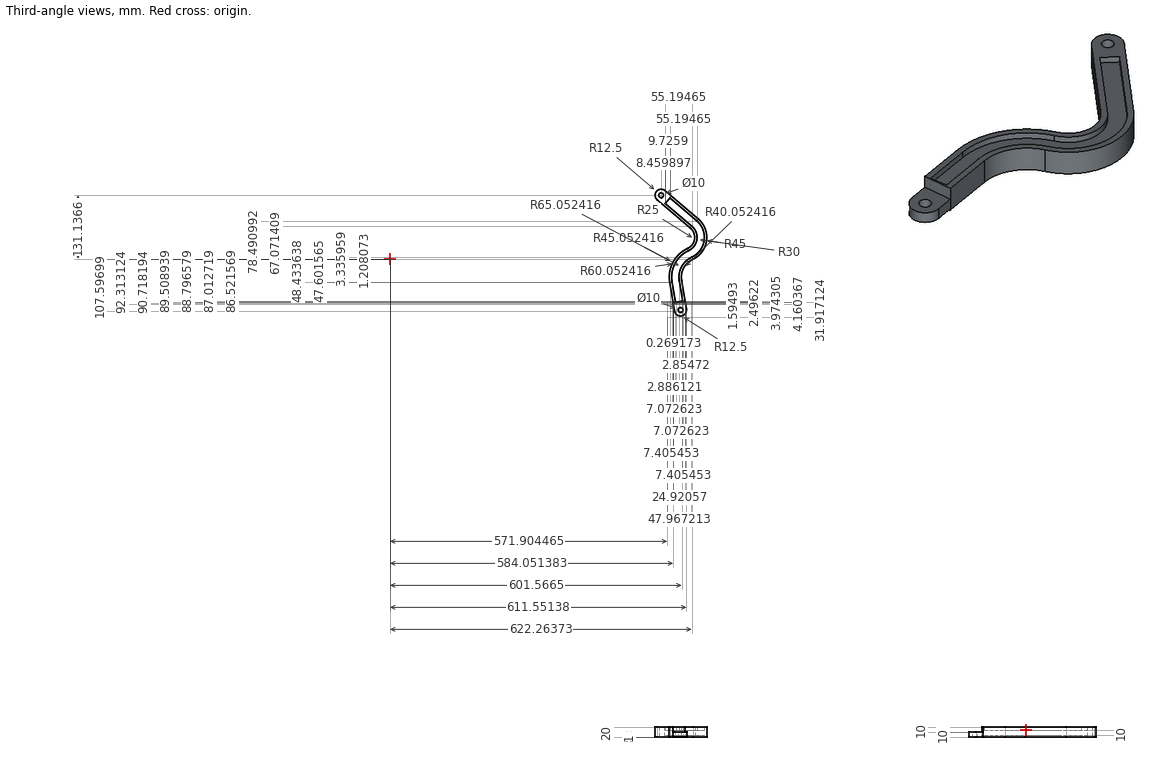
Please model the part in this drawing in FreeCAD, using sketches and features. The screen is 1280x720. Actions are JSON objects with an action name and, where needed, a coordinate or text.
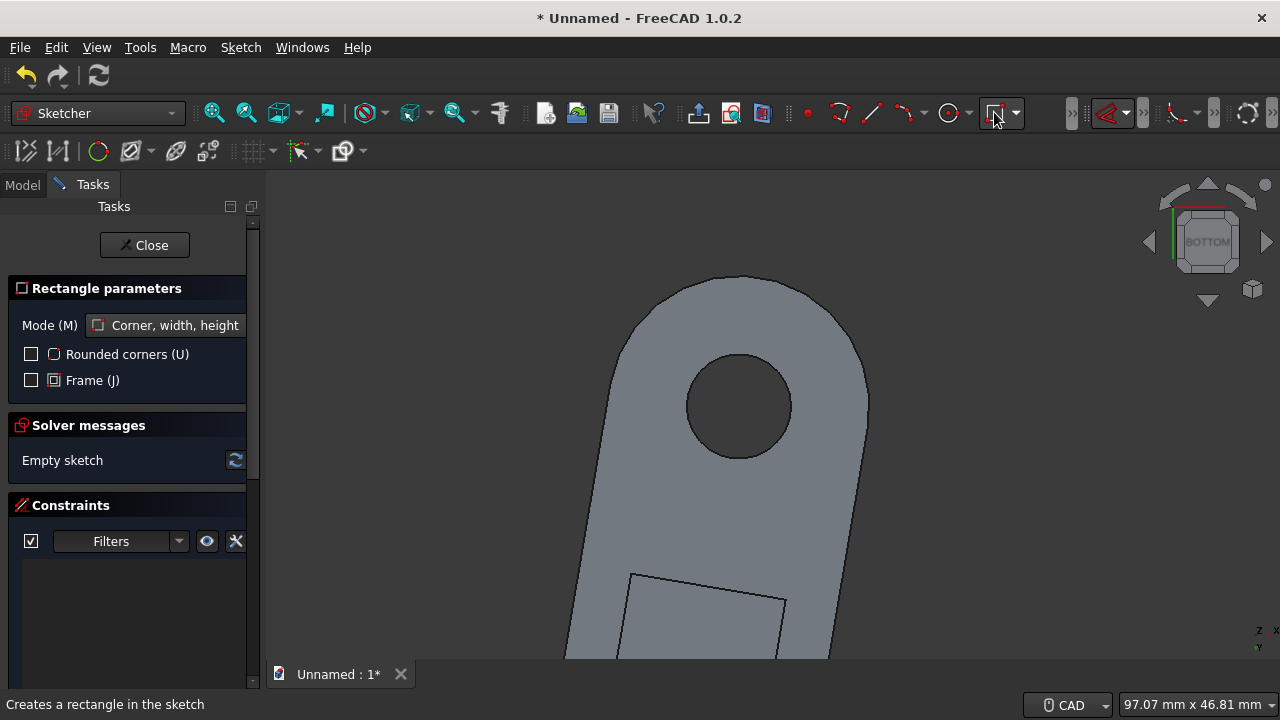
{"action": "left_click", "coordinate": [454, 248]}
{"action": "left_click", "coordinate": [955, 581]}
{"action": "key", "text": "Escape"}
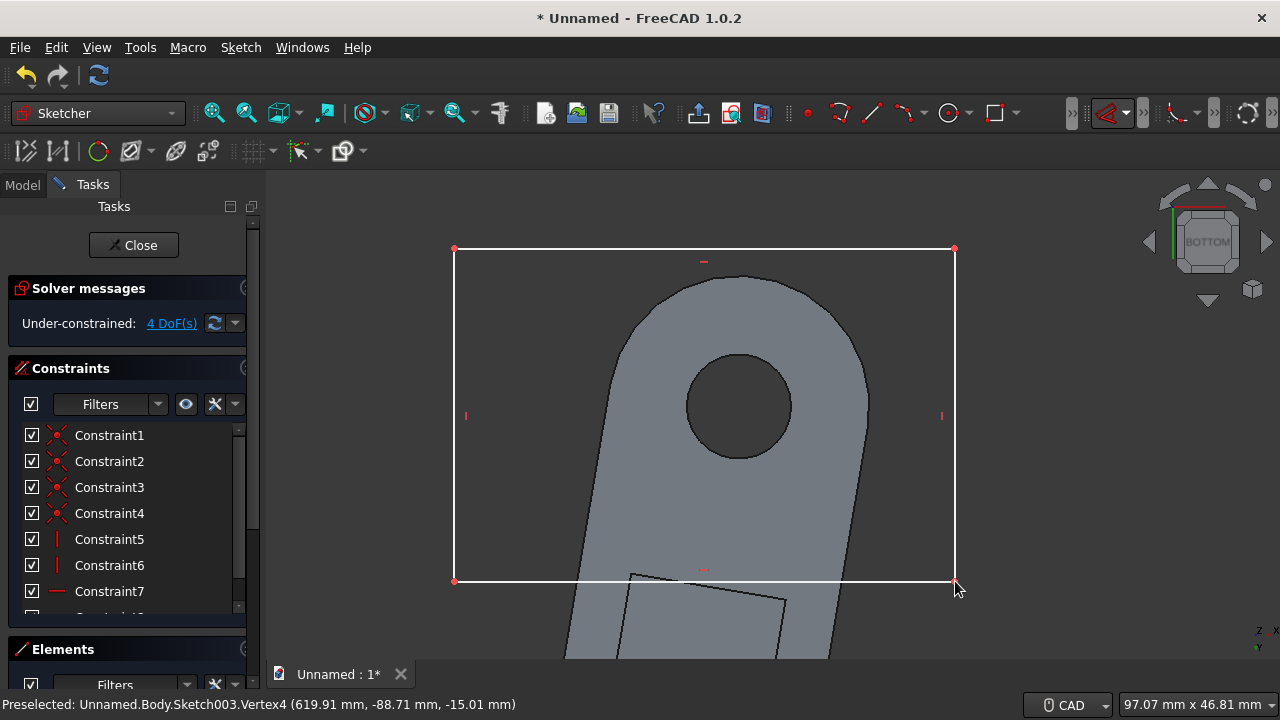
{"action": "left_click", "coordinate": [454, 349]}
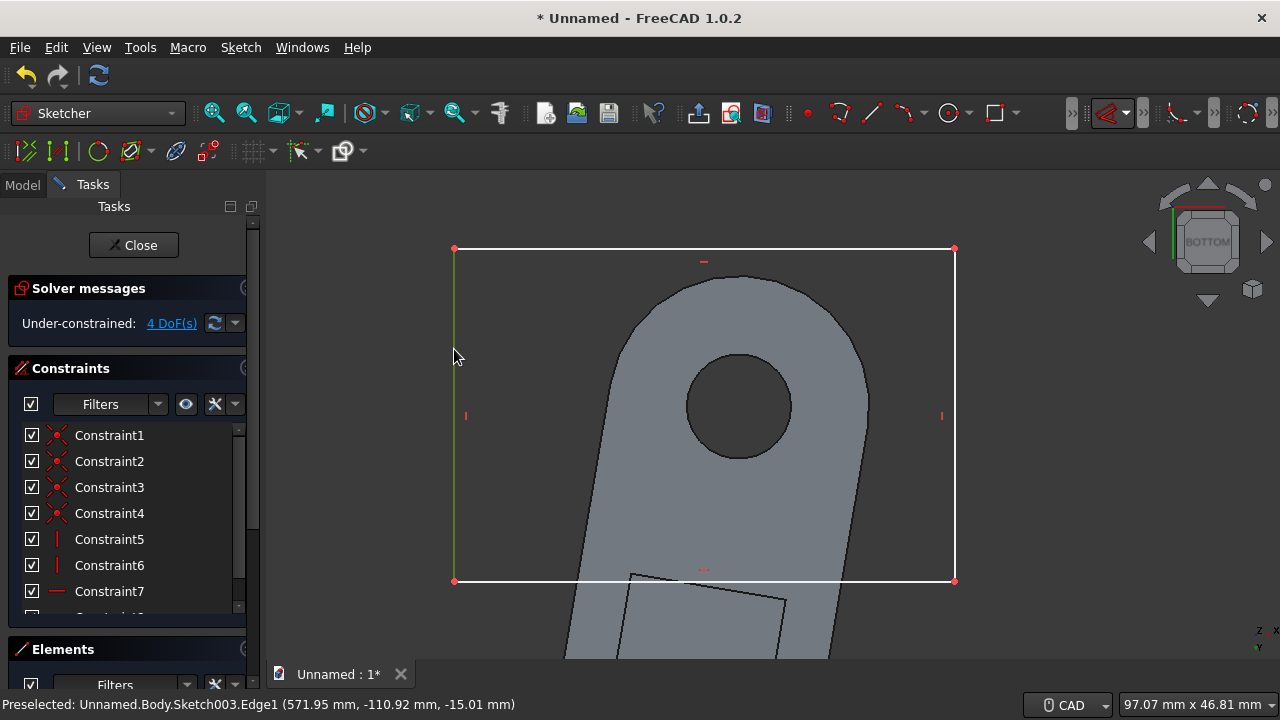
{"action": "key", "text": "i"}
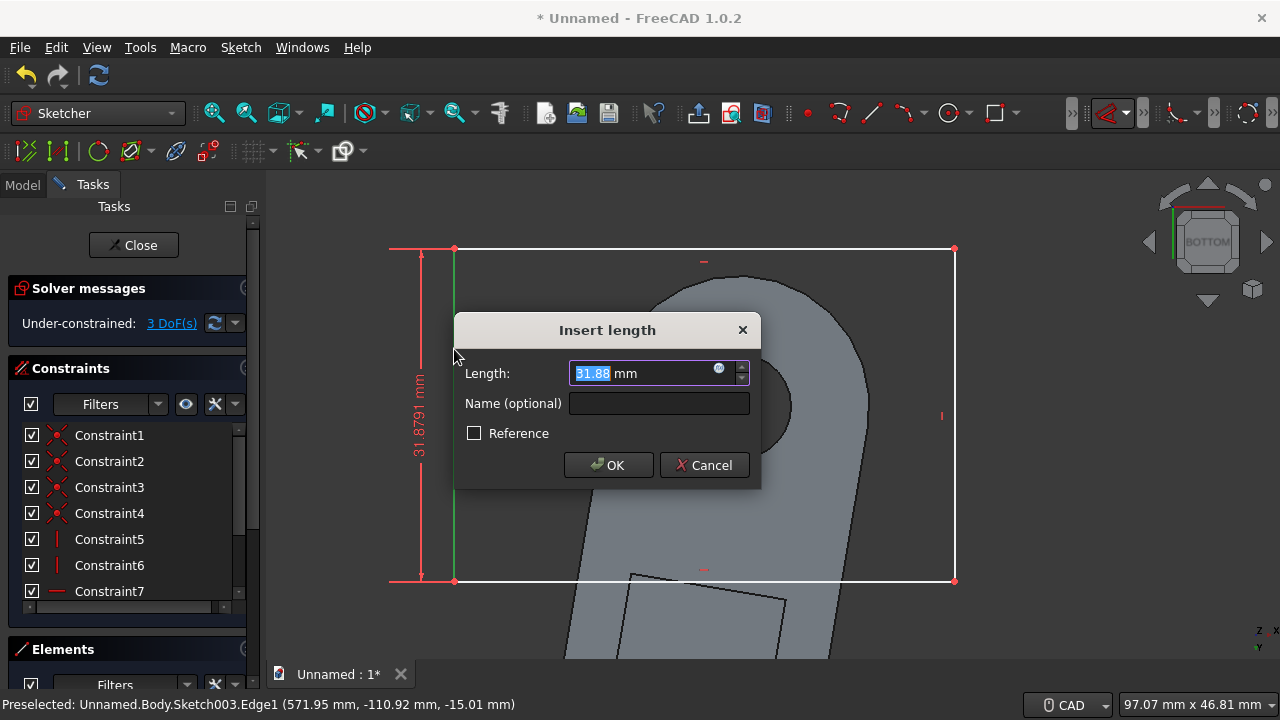
{"action": "type", "text": "31.917124"}
{"action": "key", "text": "Return"}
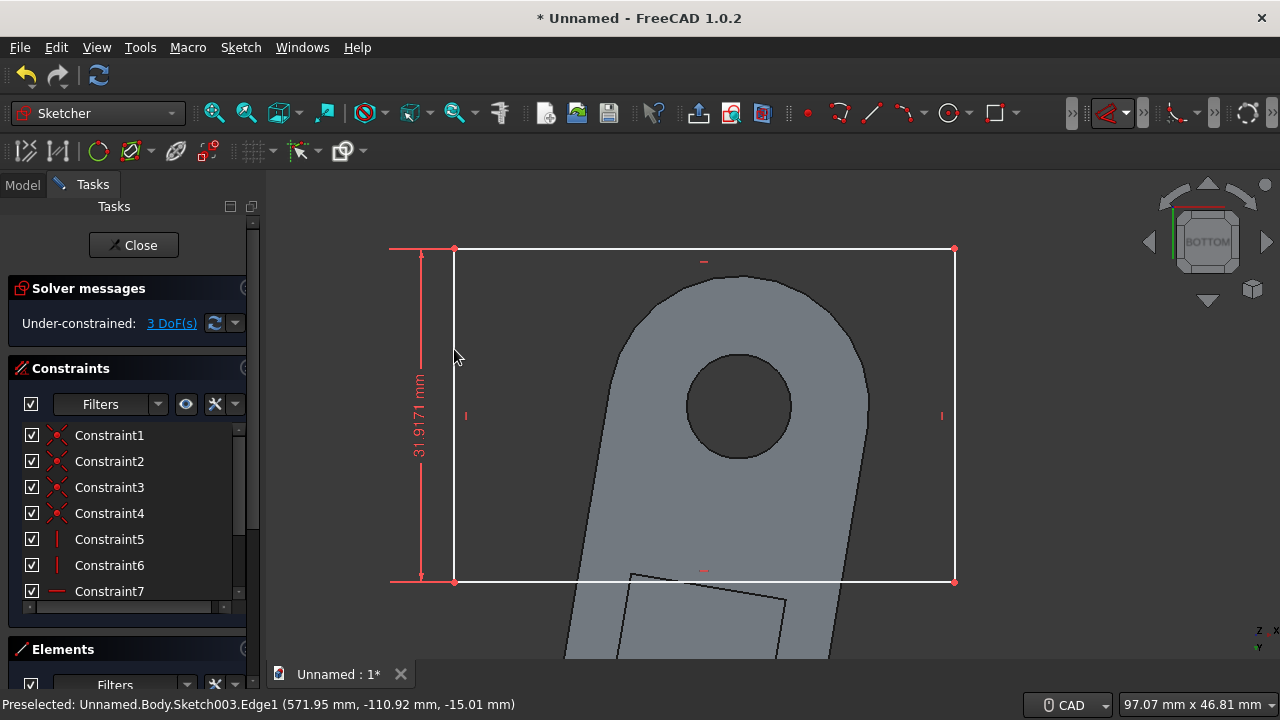
{"action": "left_click", "coordinate": [604, 582]}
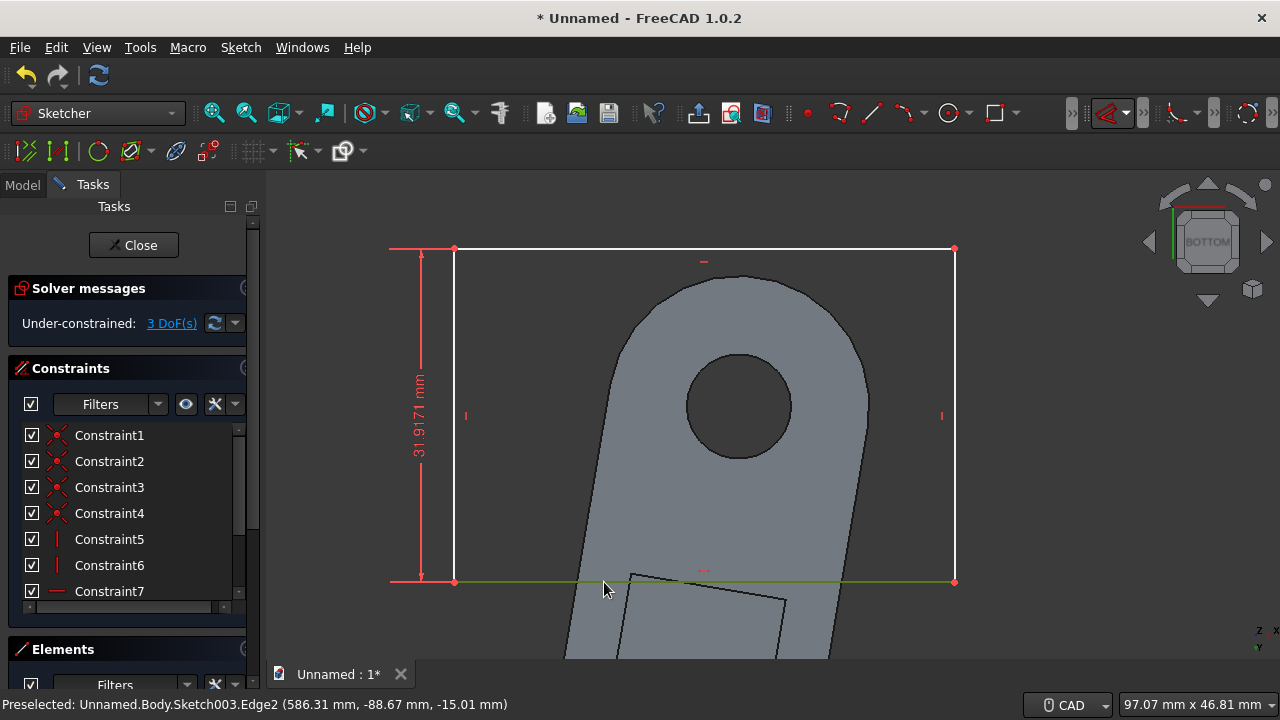
{"action": "left_click", "coordinate": [1128, 114]}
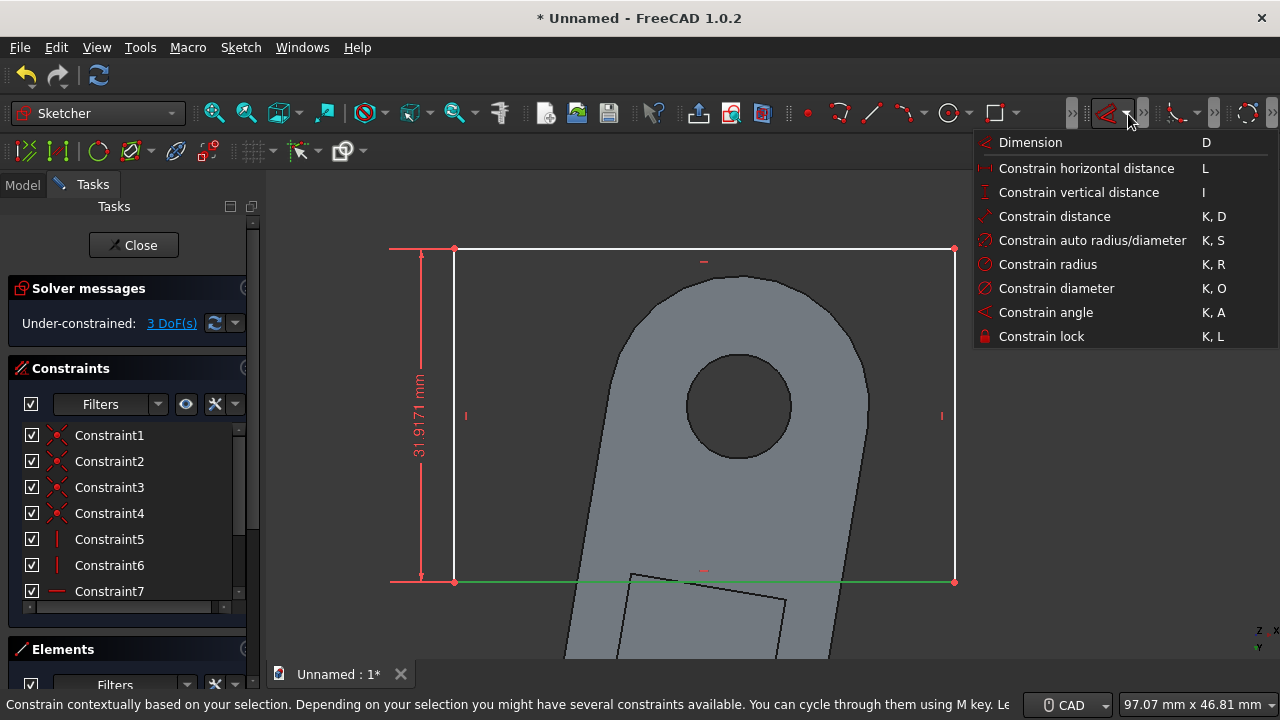
{"action": "left_click", "coordinate": [1126, 168]}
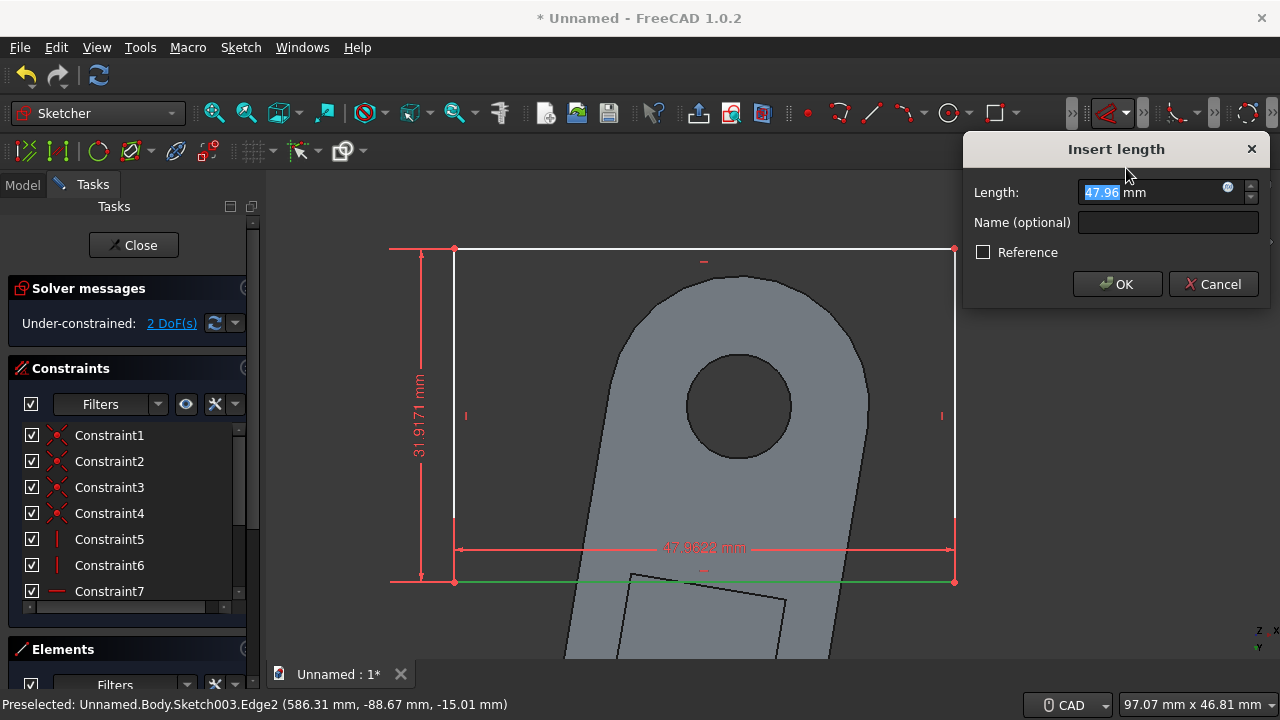
{"action": "type", "text": "47.967213"}
{"action": "key", "text": "Return"}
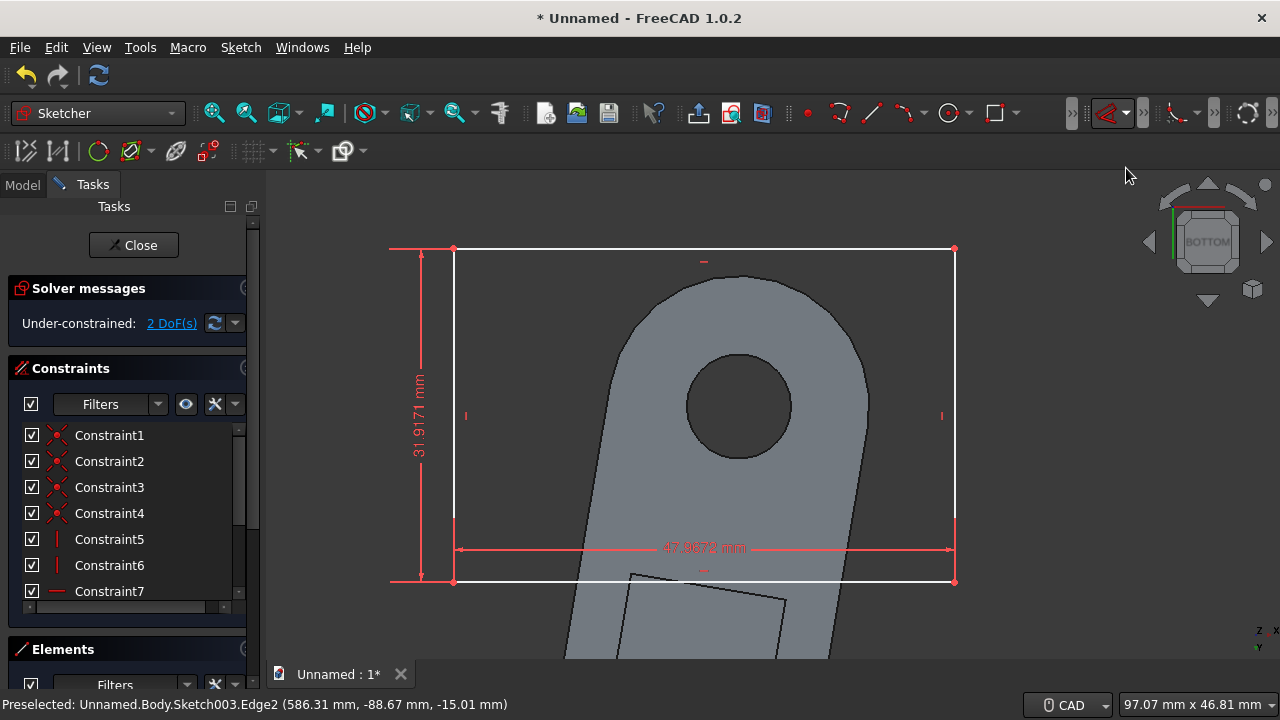
{"action": "left_click", "coordinate": [454, 582]}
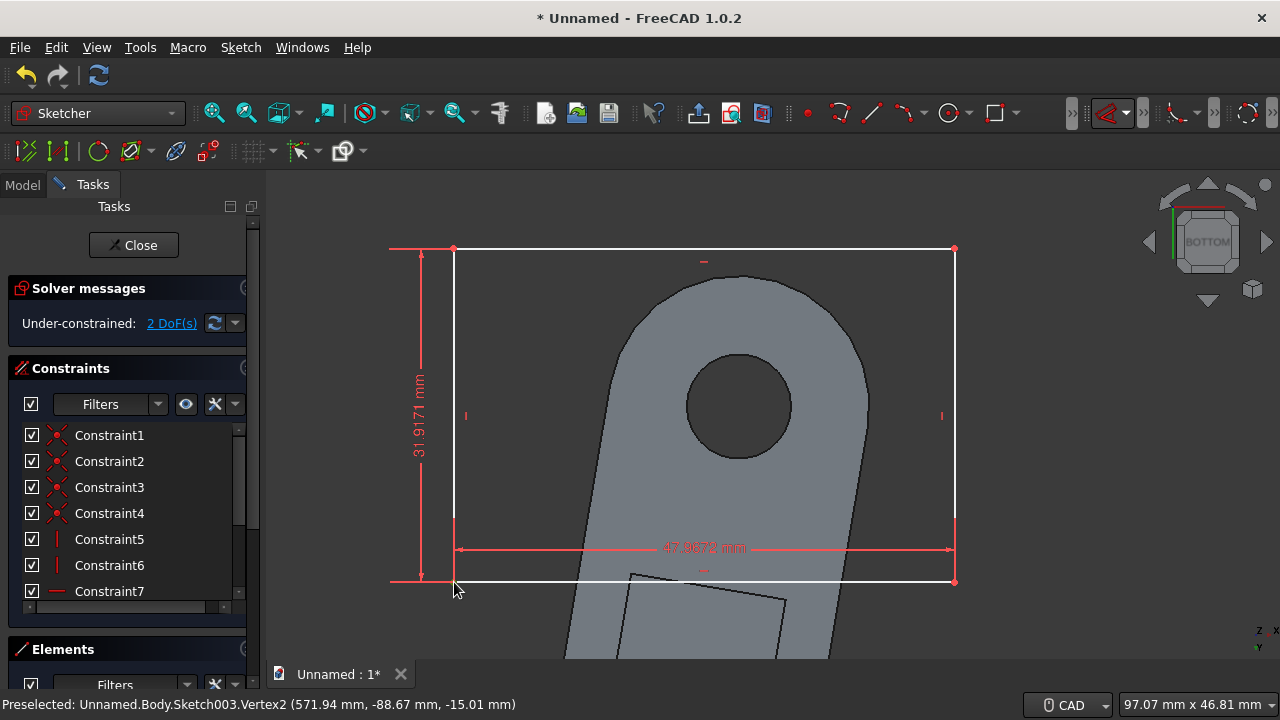
{"action": "left_click", "coordinate": [1128, 114]}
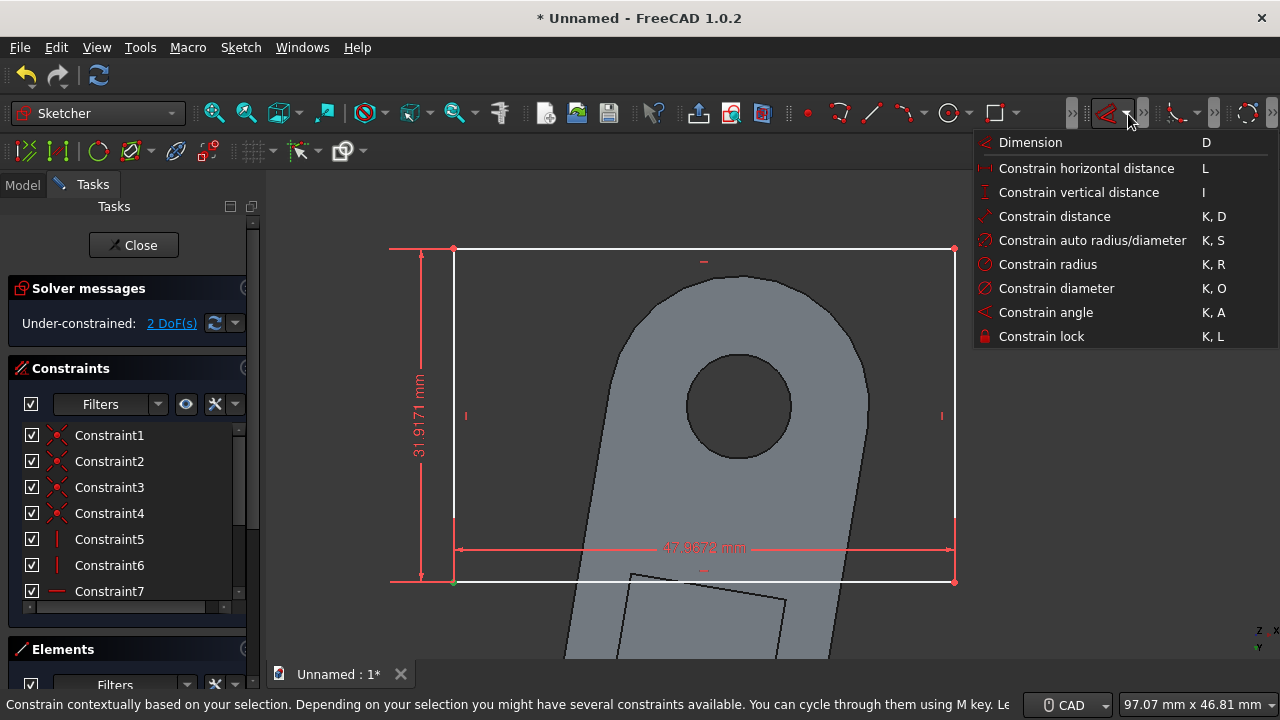
{"action": "left_click", "coordinate": [1126, 192]}